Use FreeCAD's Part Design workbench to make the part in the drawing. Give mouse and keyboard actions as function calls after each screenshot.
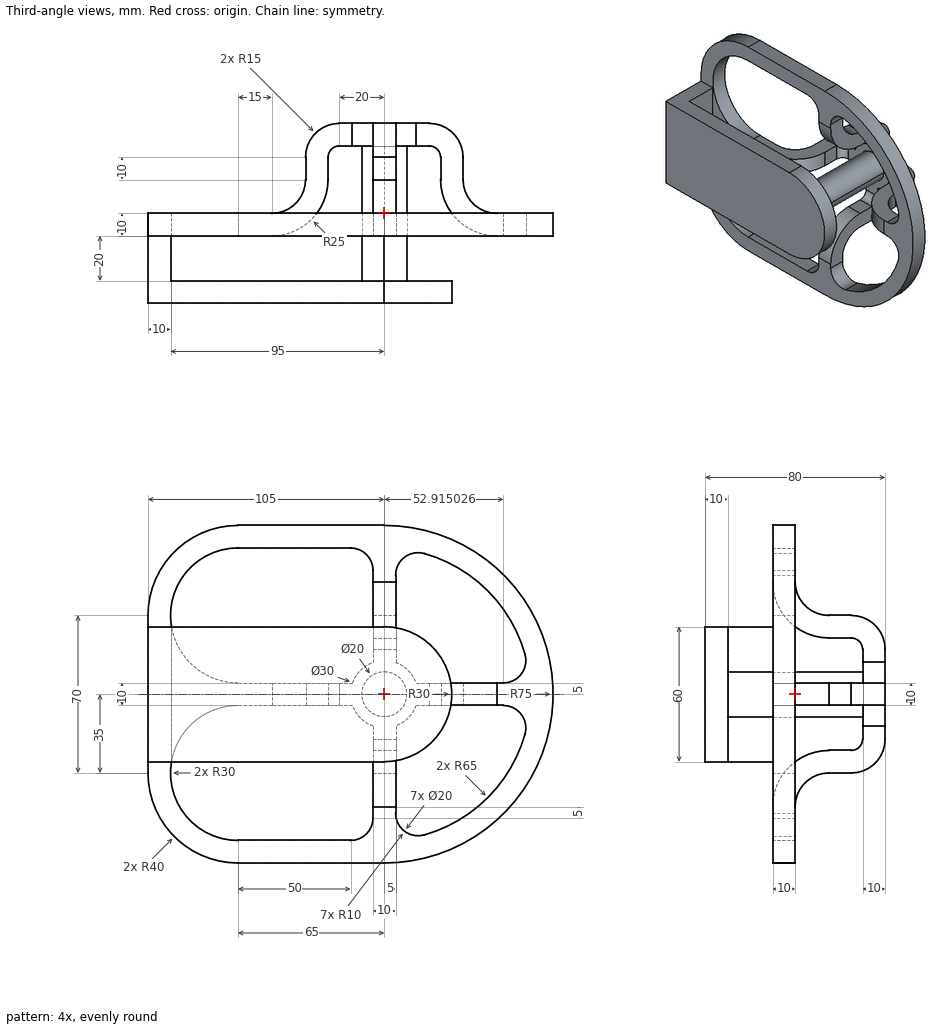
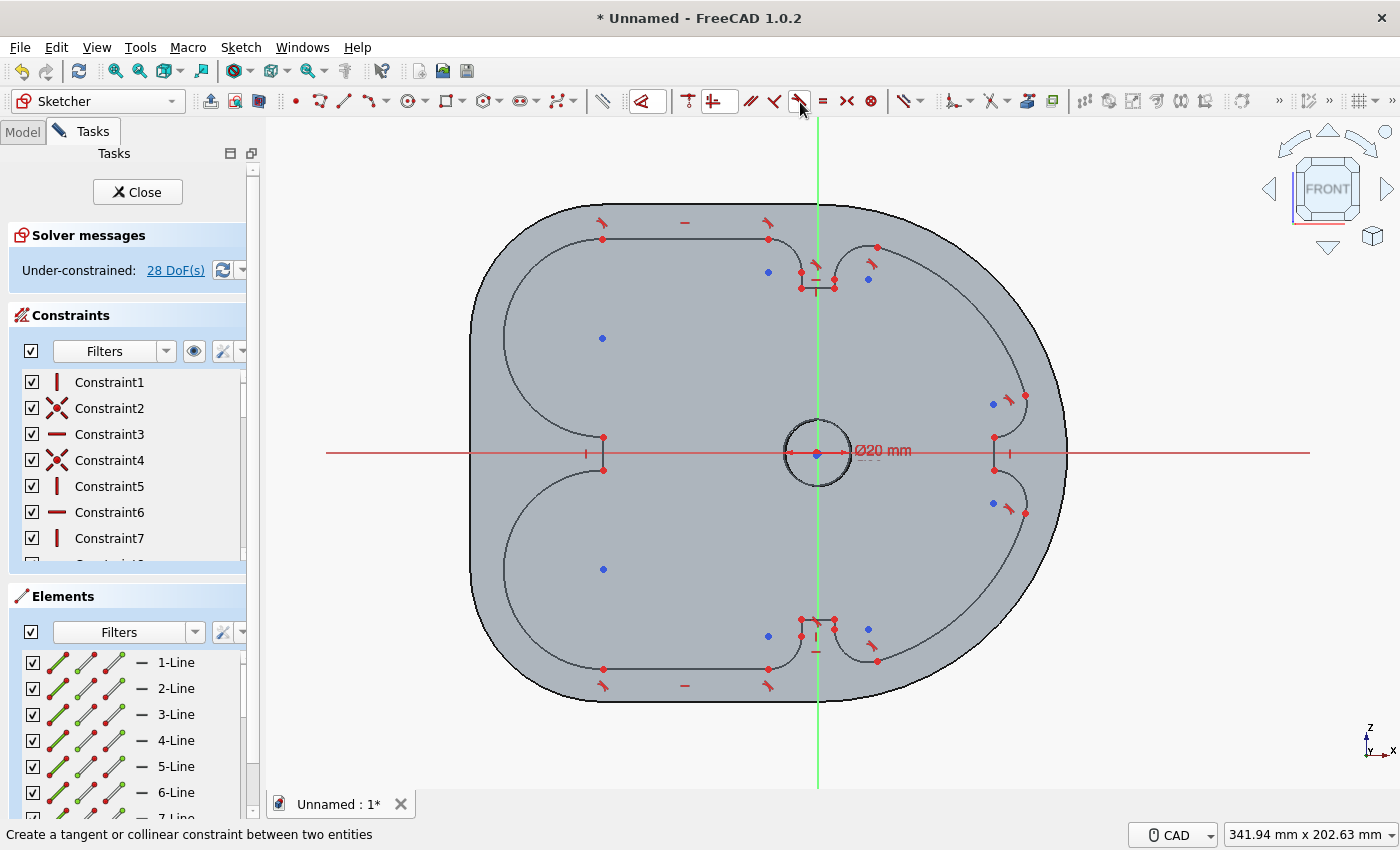
click(840, 429)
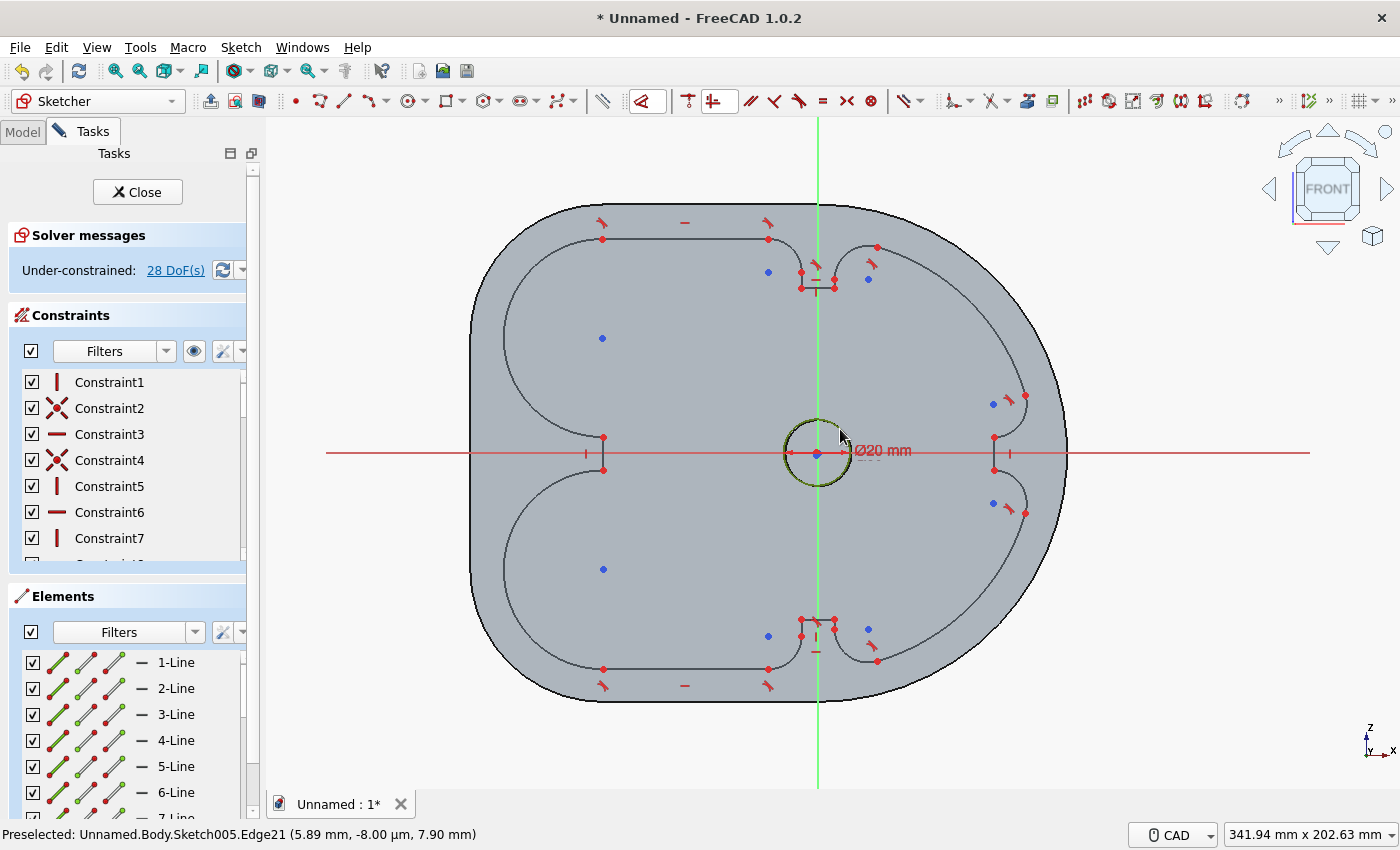
click(998, 336)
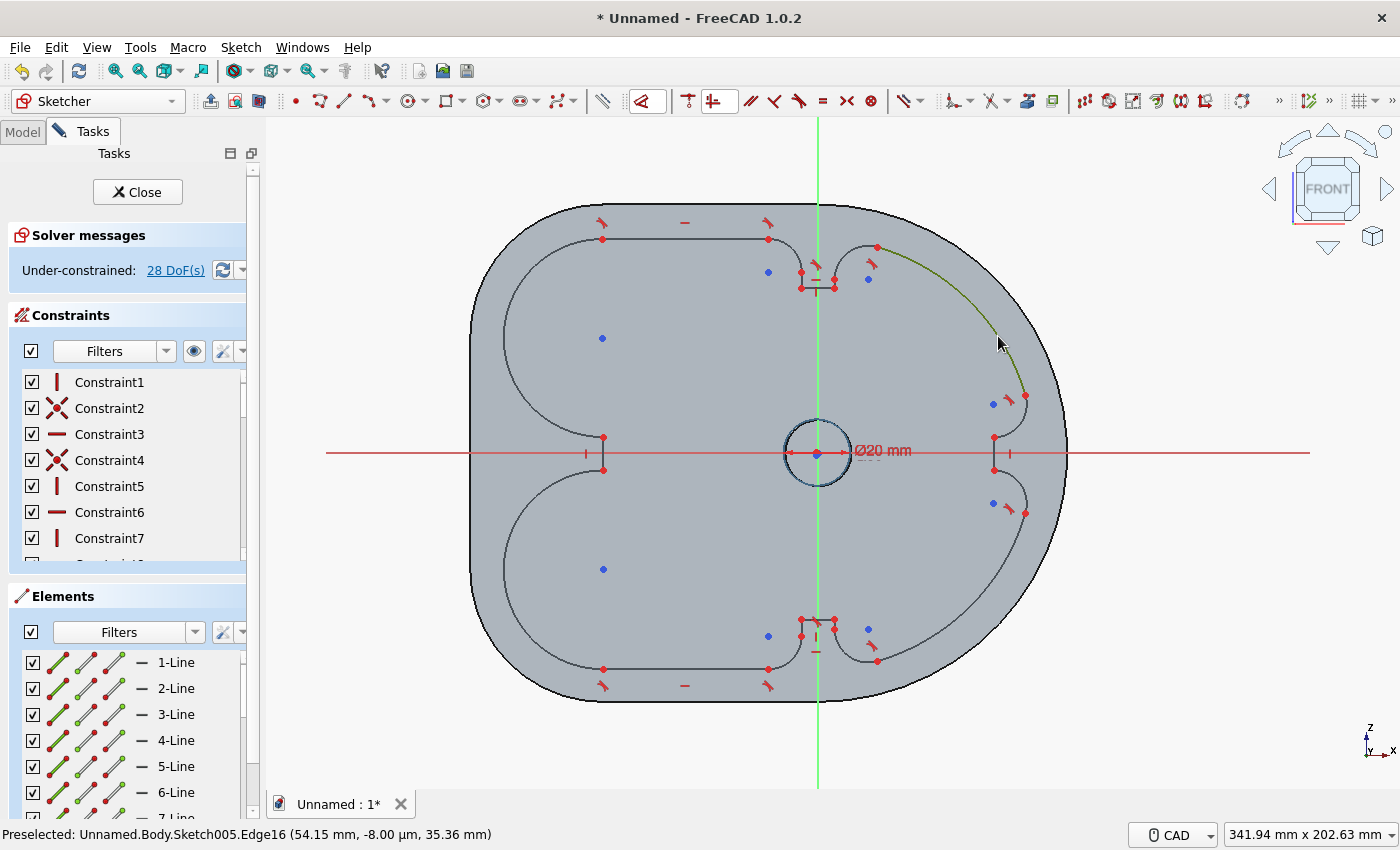
click(688, 102)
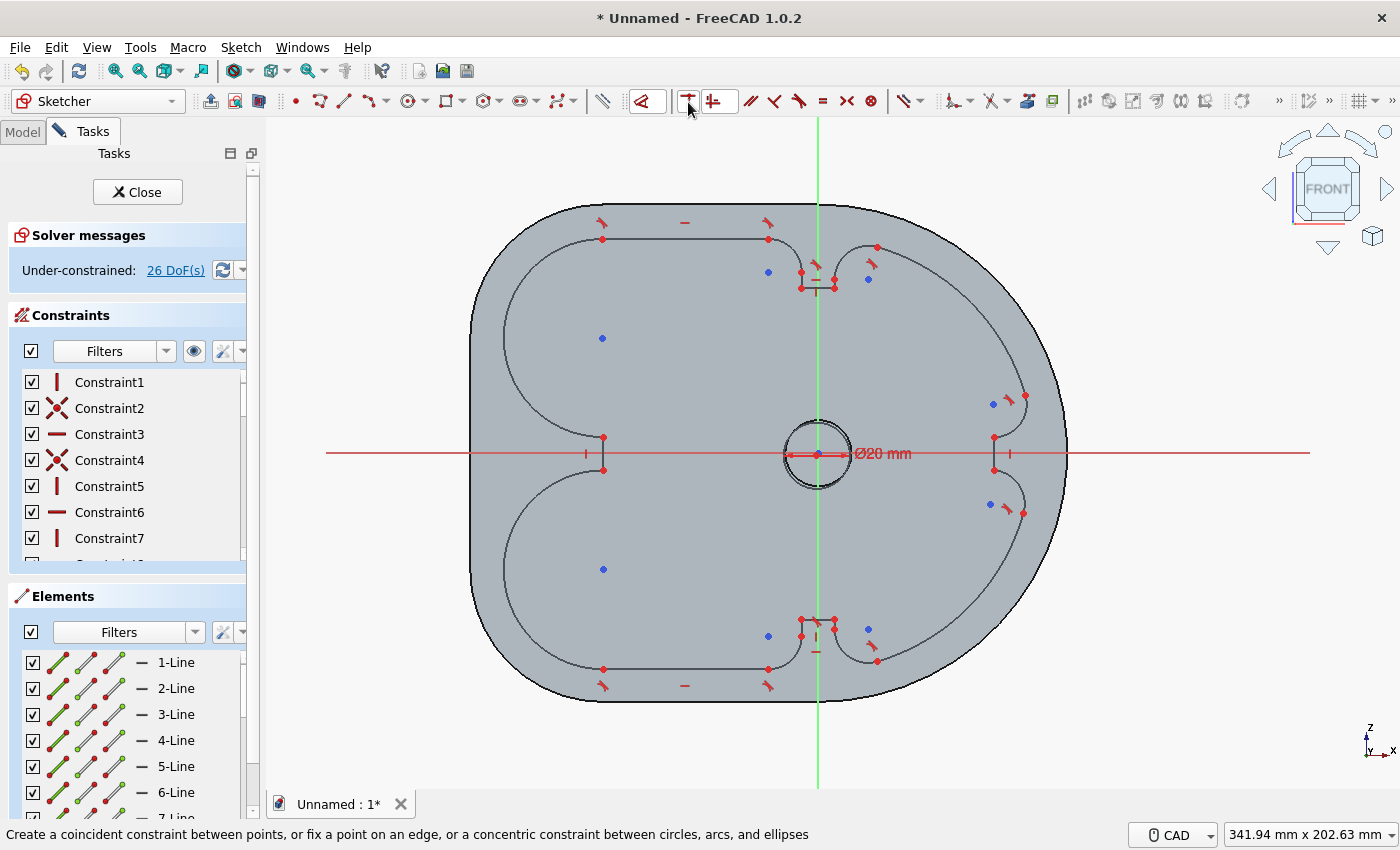
drag(807, 443, 828, 466)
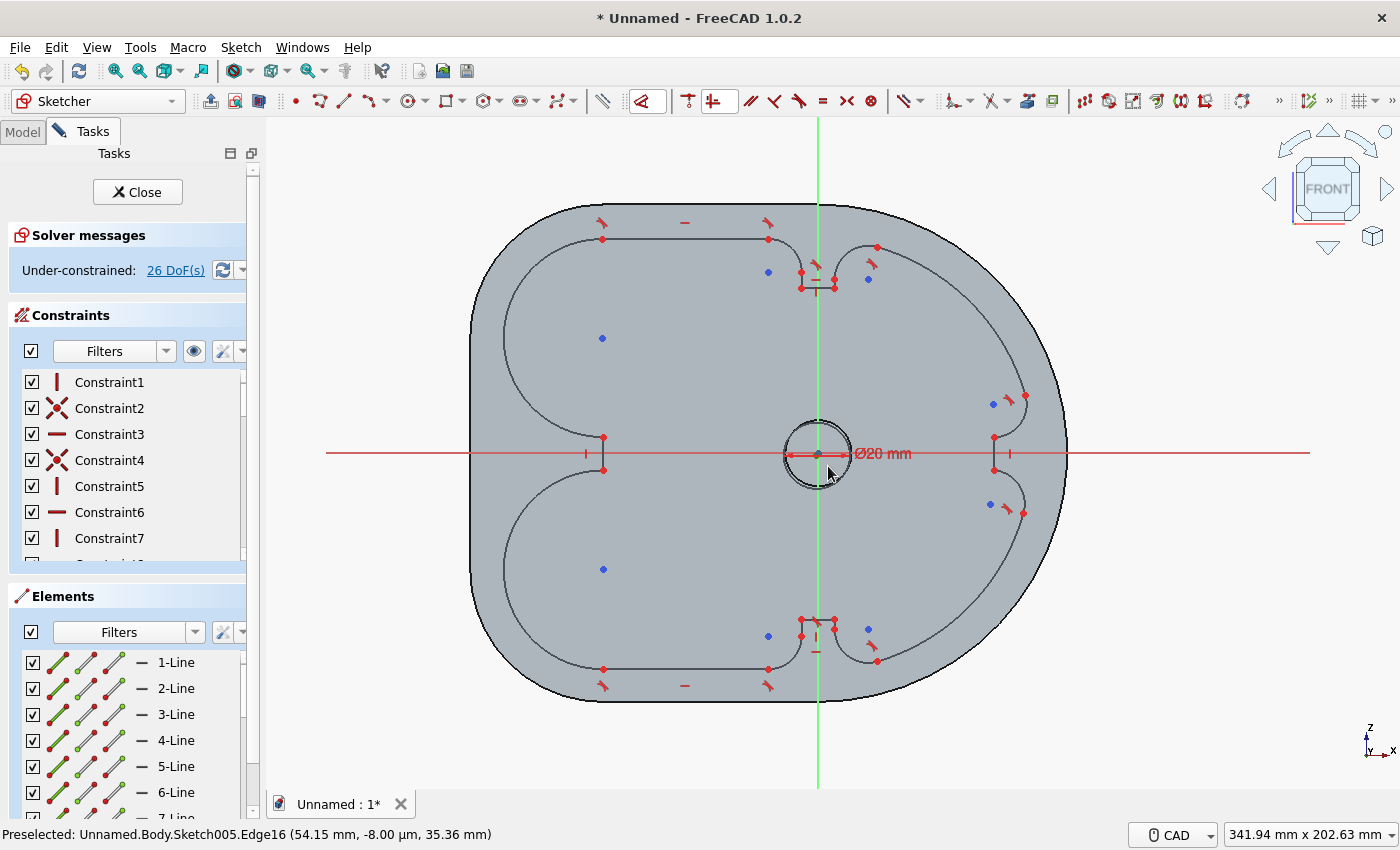
click(688, 102)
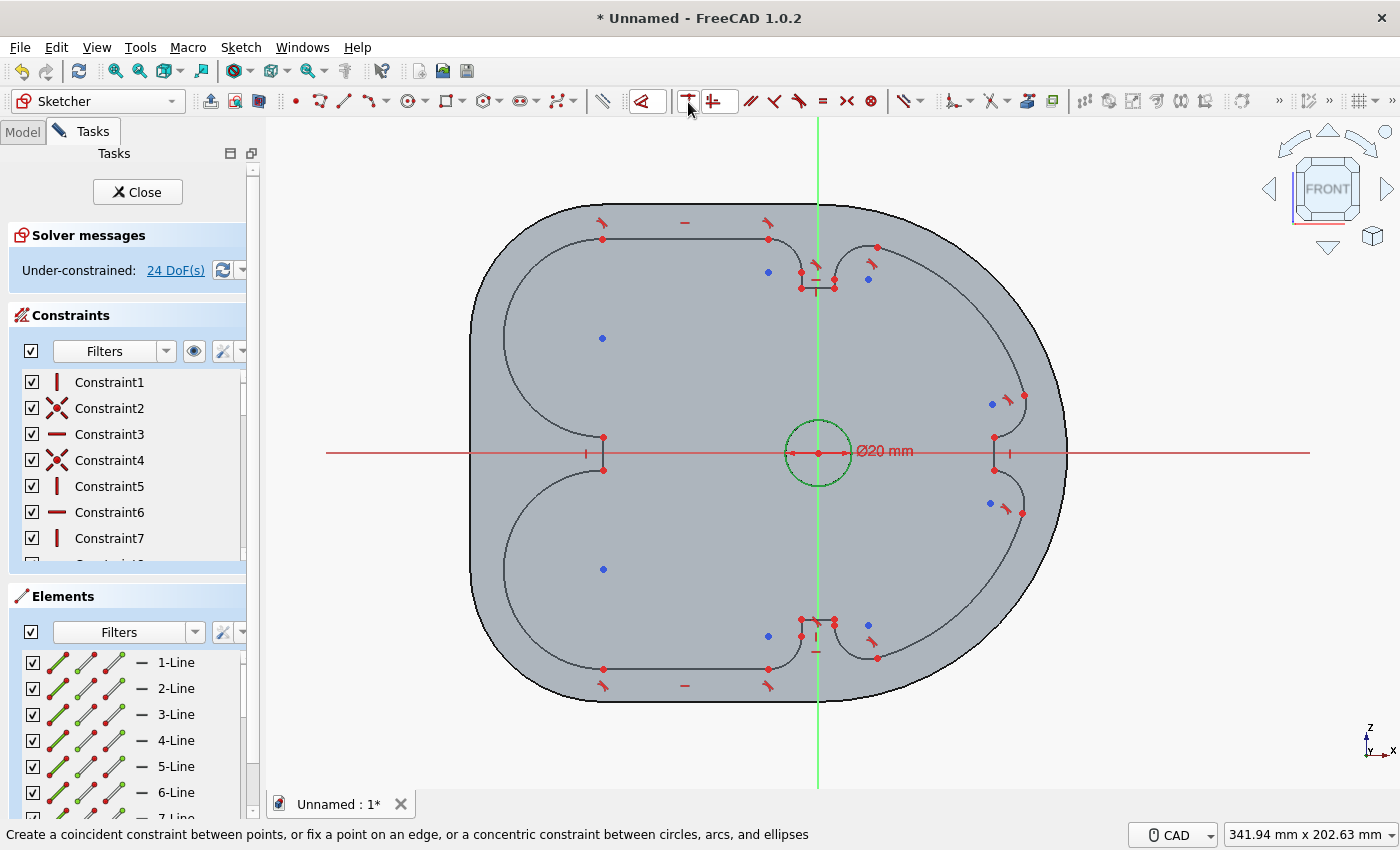
click(523, 511)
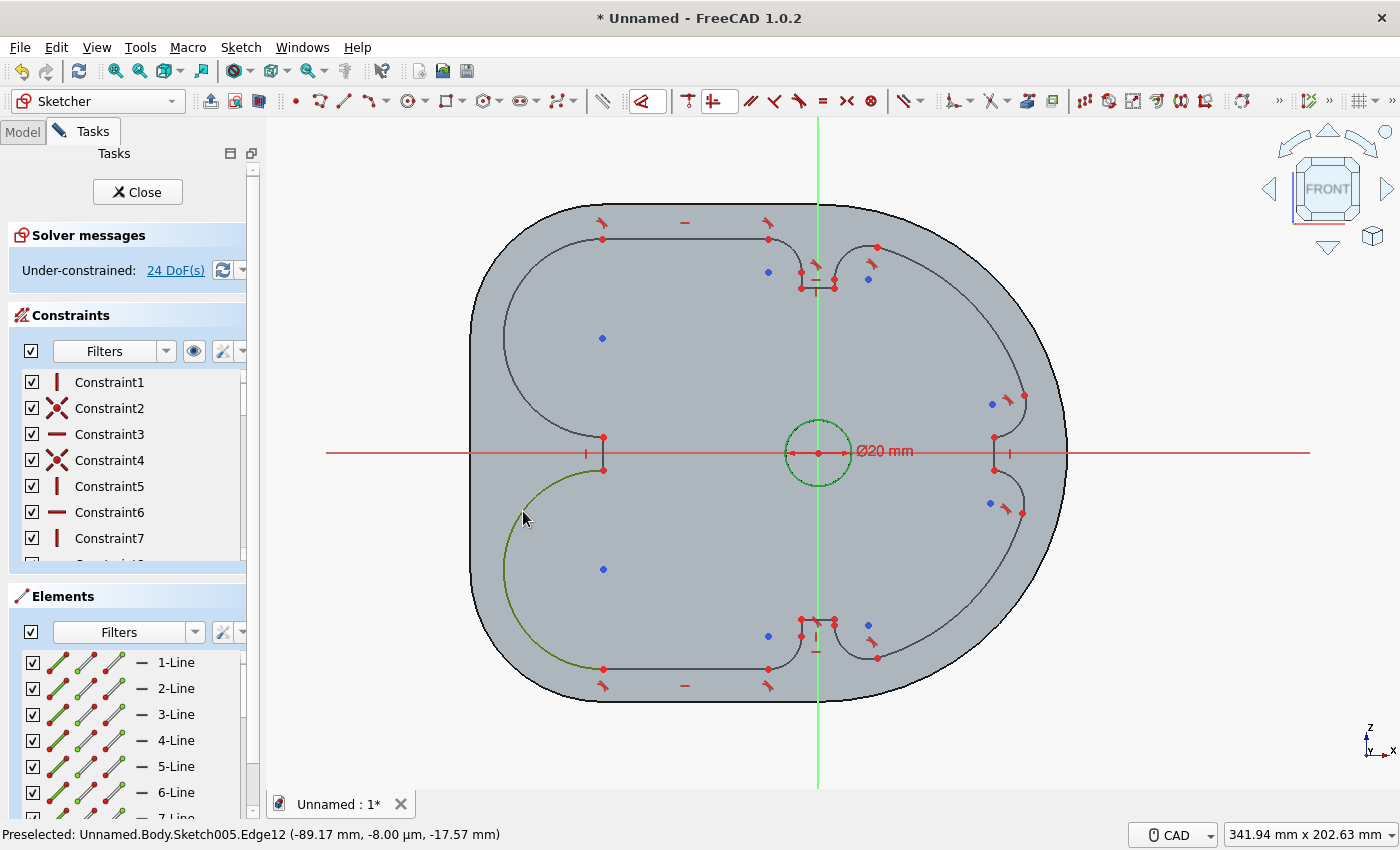
click(523, 280)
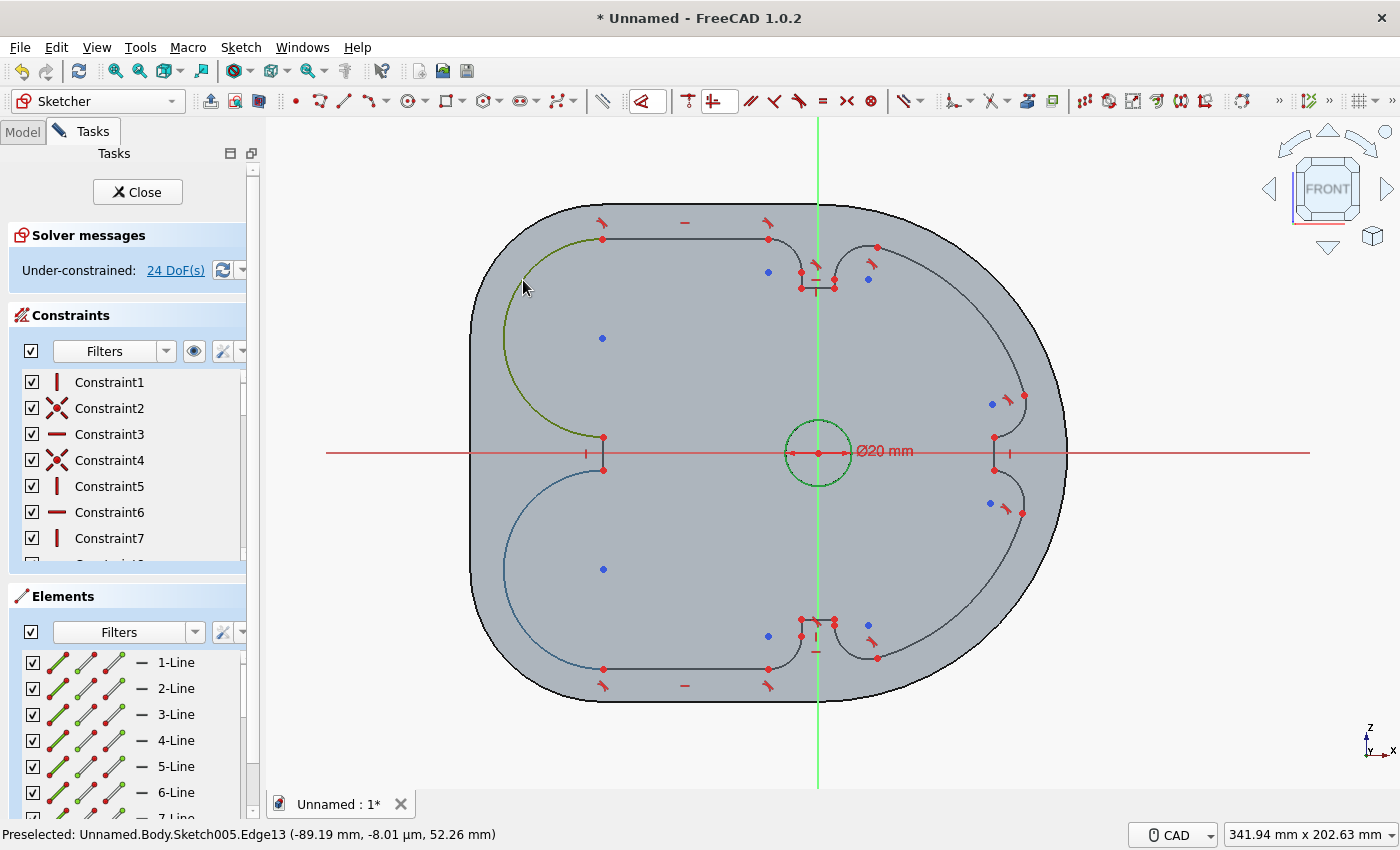
click(824, 102)